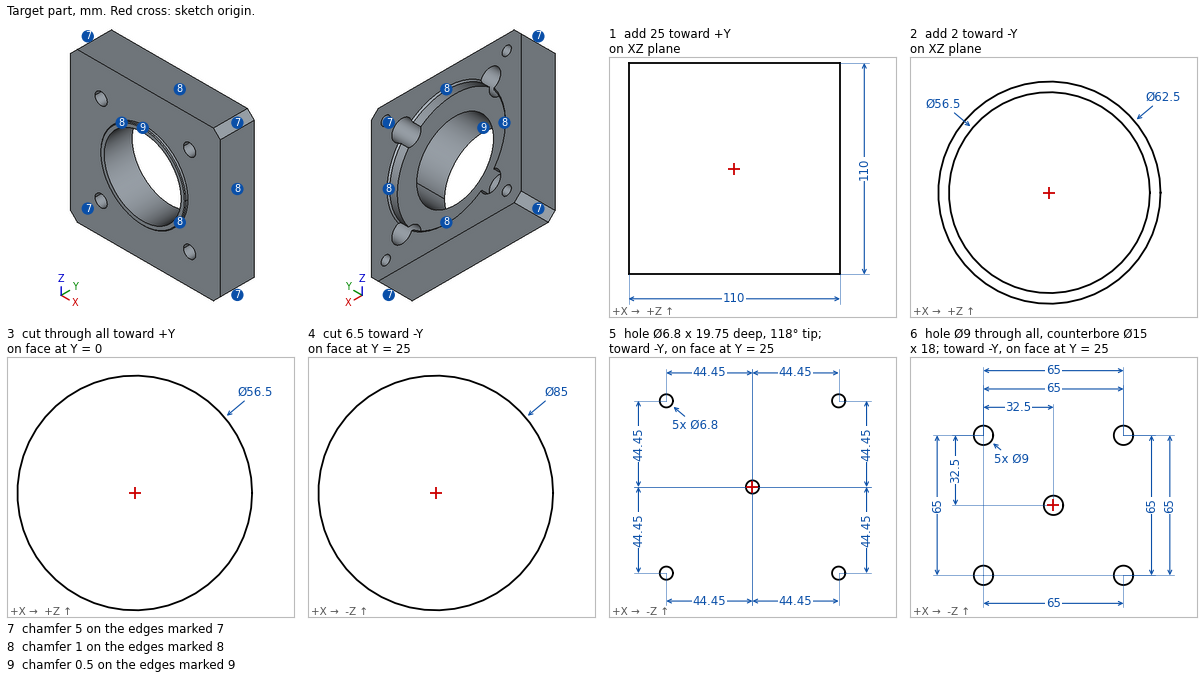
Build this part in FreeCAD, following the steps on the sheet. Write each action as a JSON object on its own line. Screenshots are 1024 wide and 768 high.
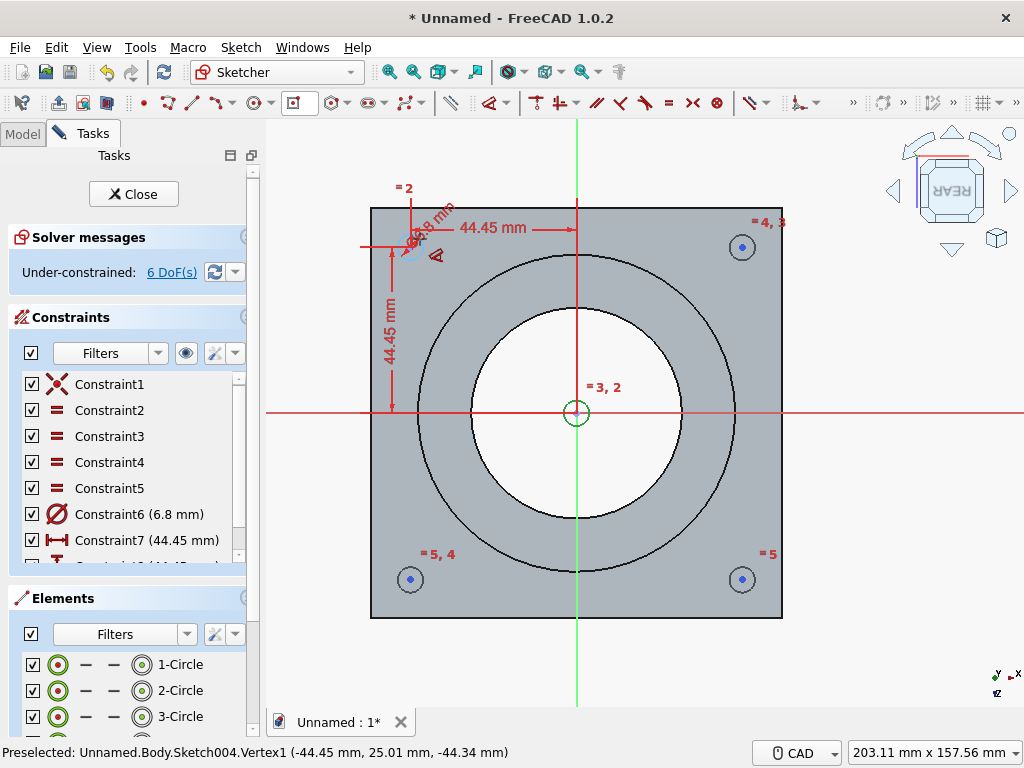
{"action": "left_click", "coordinate": [742, 248]}
{"action": "left_click", "coordinate": [659, 214]}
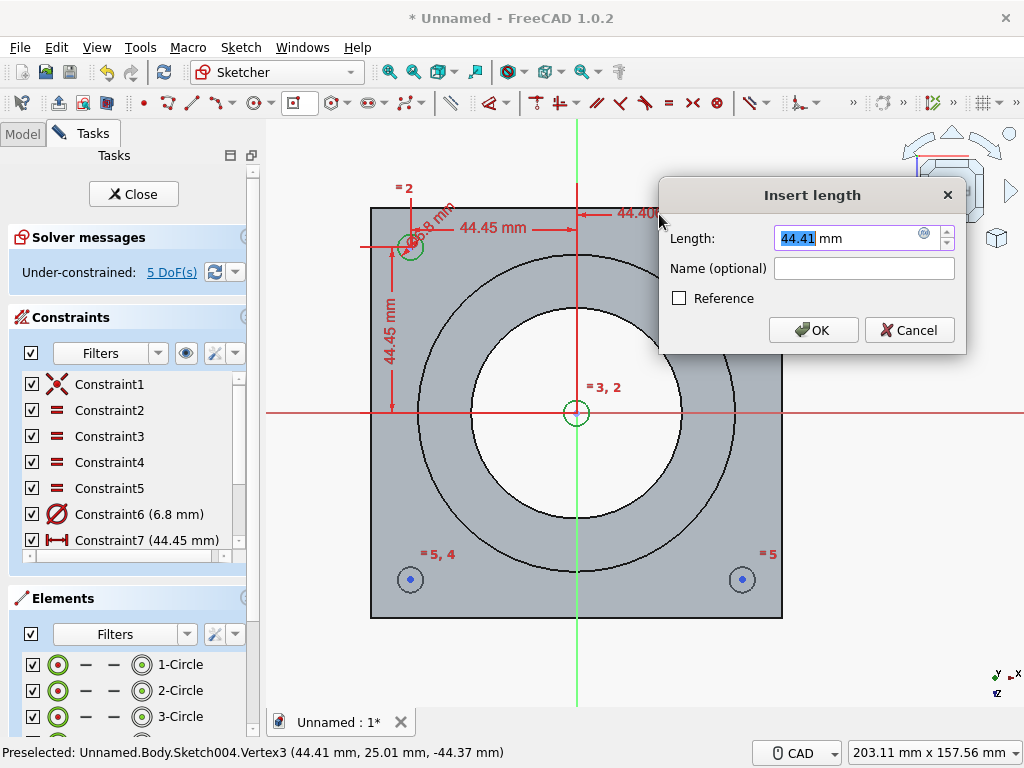
{"action": "type", "text": "44.45"}
{"action": "key", "text": "Return"}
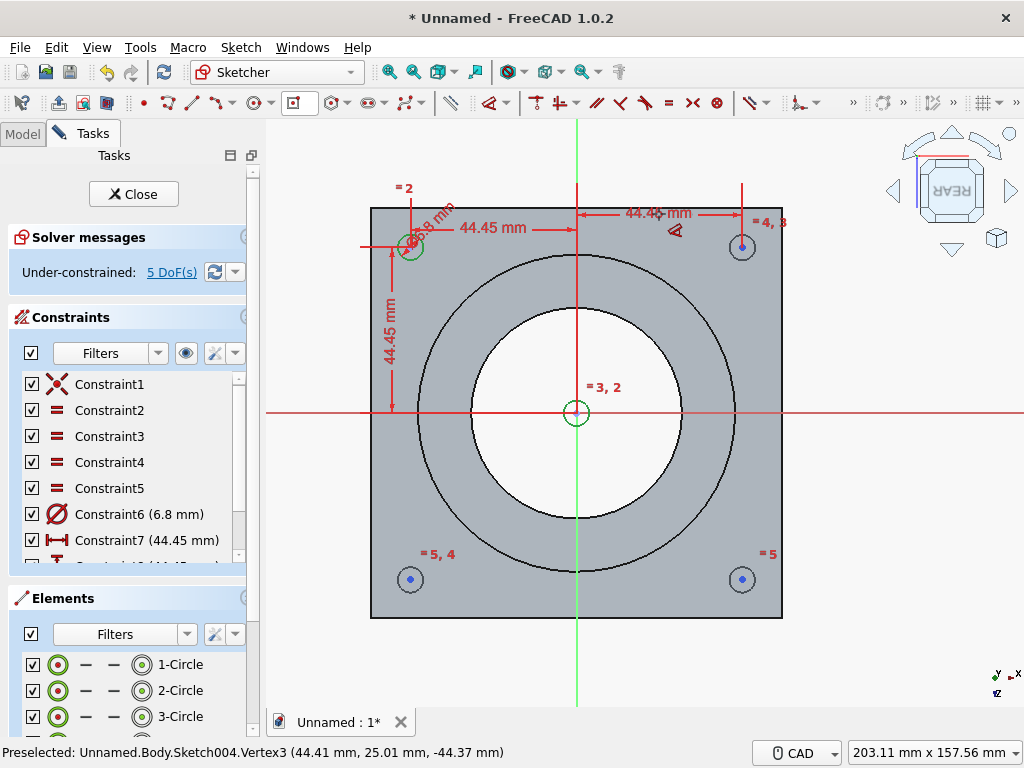
{"action": "left_click", "coordinate": [742, 248]}
{"action": "left_click", "coordinate": [776, 330]}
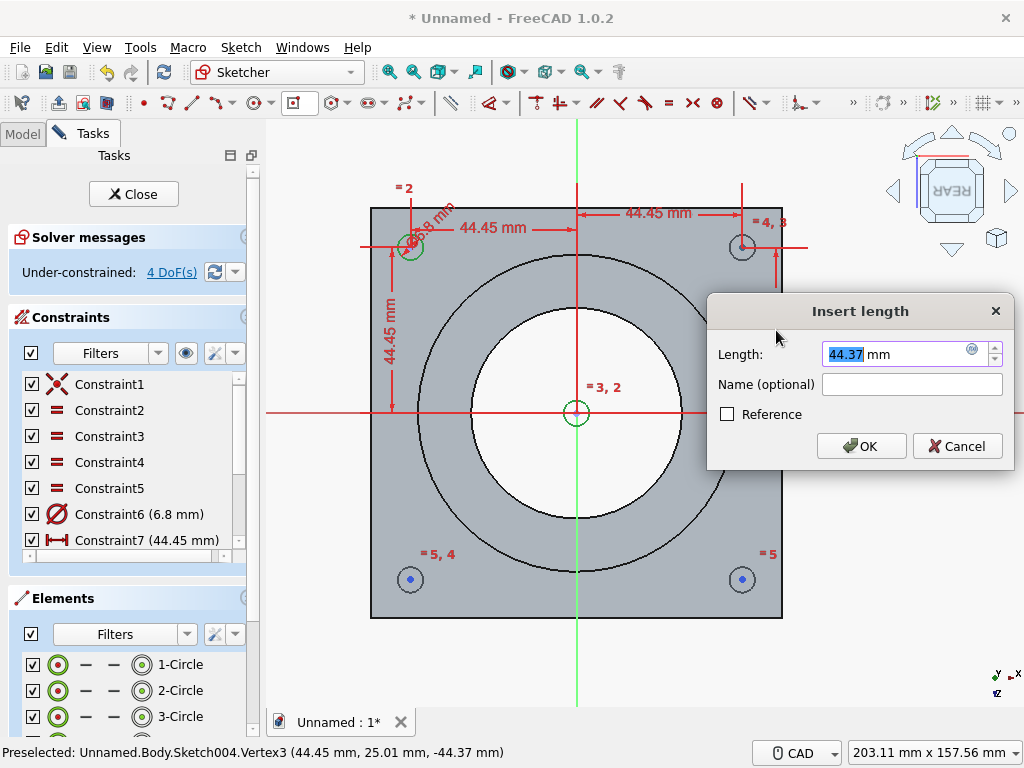
{"action": "type", "text": "44.45"}
{"action": "key", "text": "Return"}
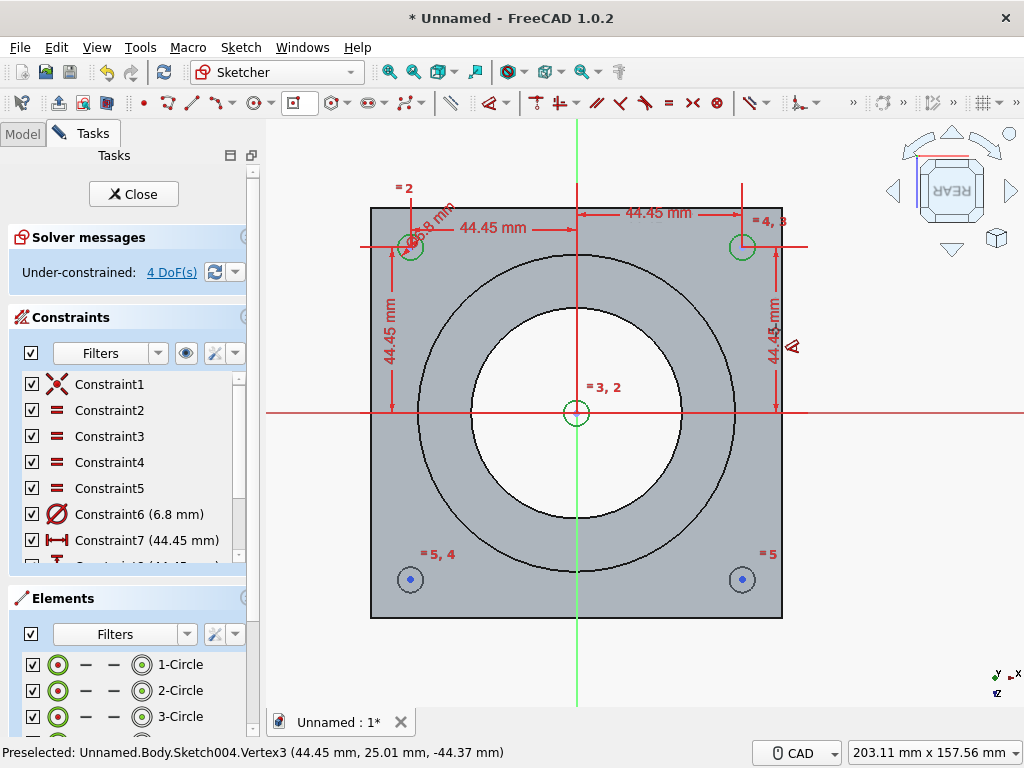
{"action": "left_click", "coordinate": [411, 580]}
{"action": "left_click", "coordinate": [494, 614]}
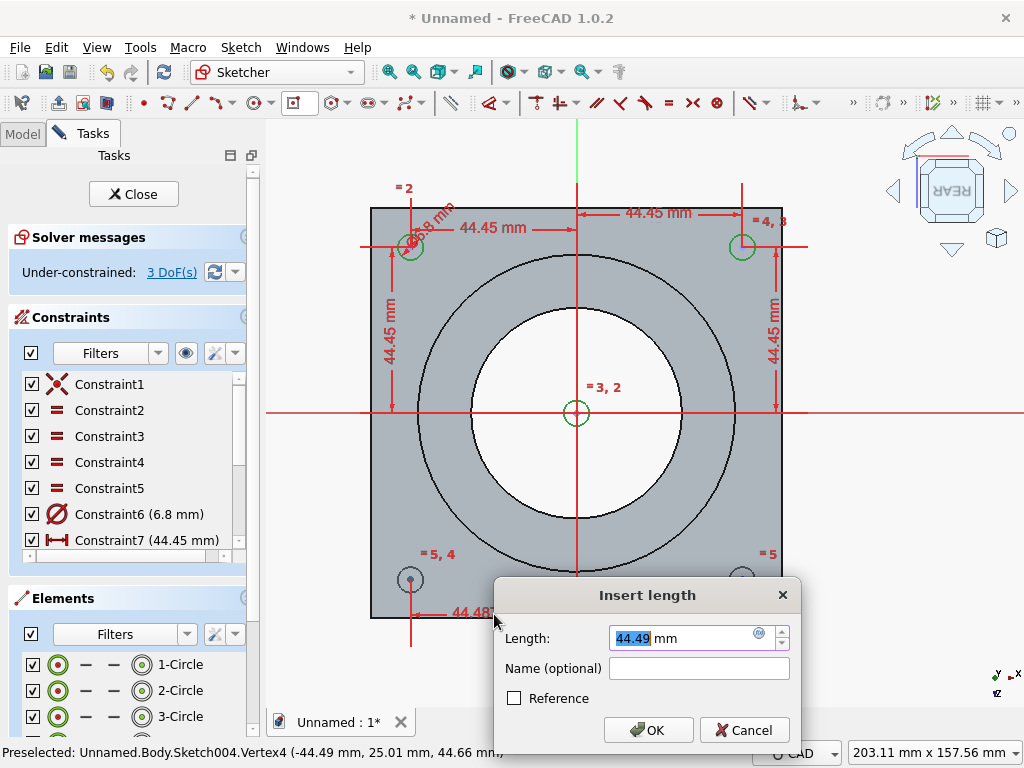
{"action": "type", "text": "44.45"}
{"action": "key", "text": "Return"}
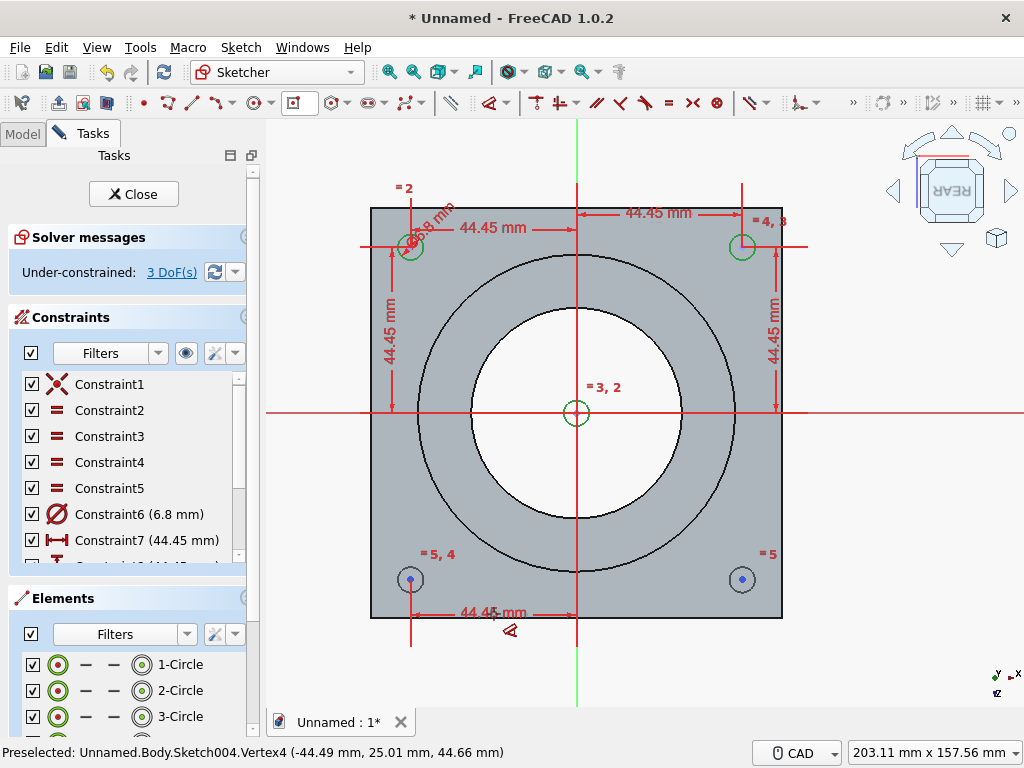
{"action": "left_click", "coordinate": [411, 580]}
{"action": "left_click", "coordinate": [377, 497]}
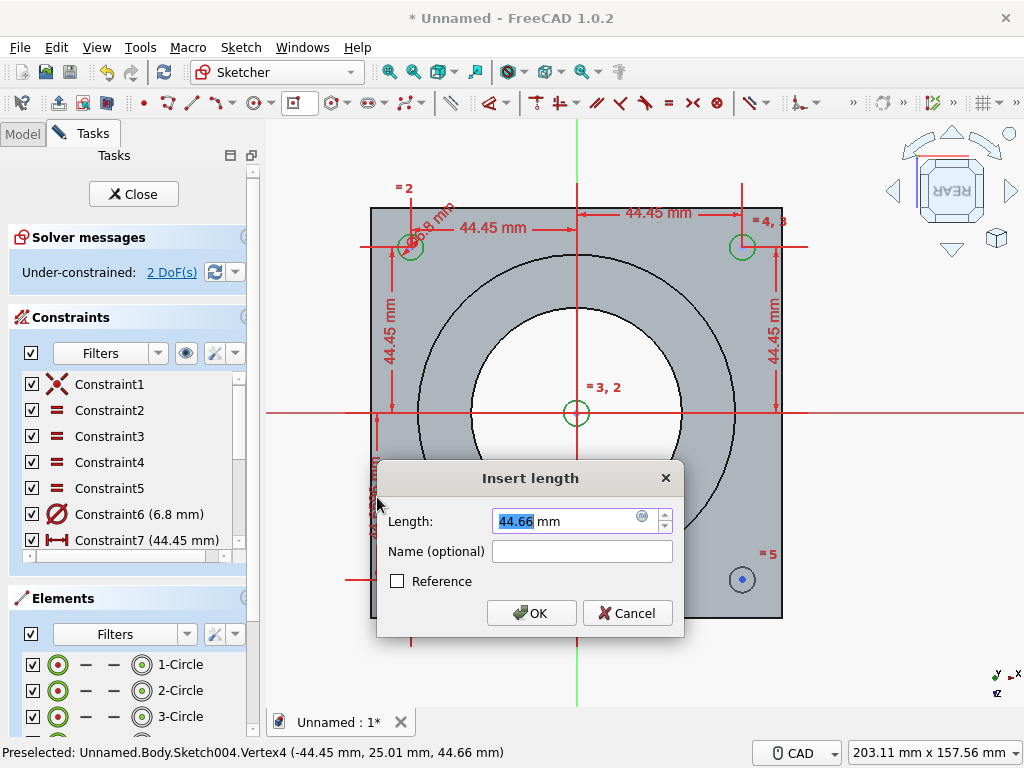
{"action": "type", "text": "44.45"}
{"action": "key", "text": "Return"}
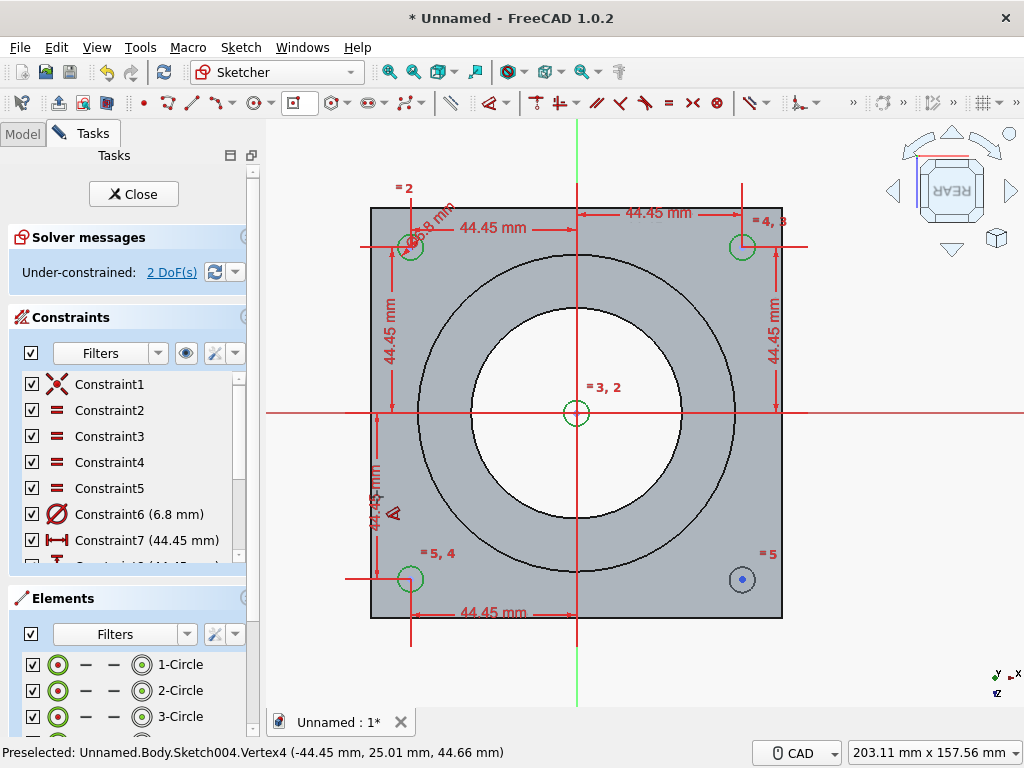
{"action": "left_click", "coordinate": [742, 580]}
{"action": "left_click", "coordinate": [659, 614]}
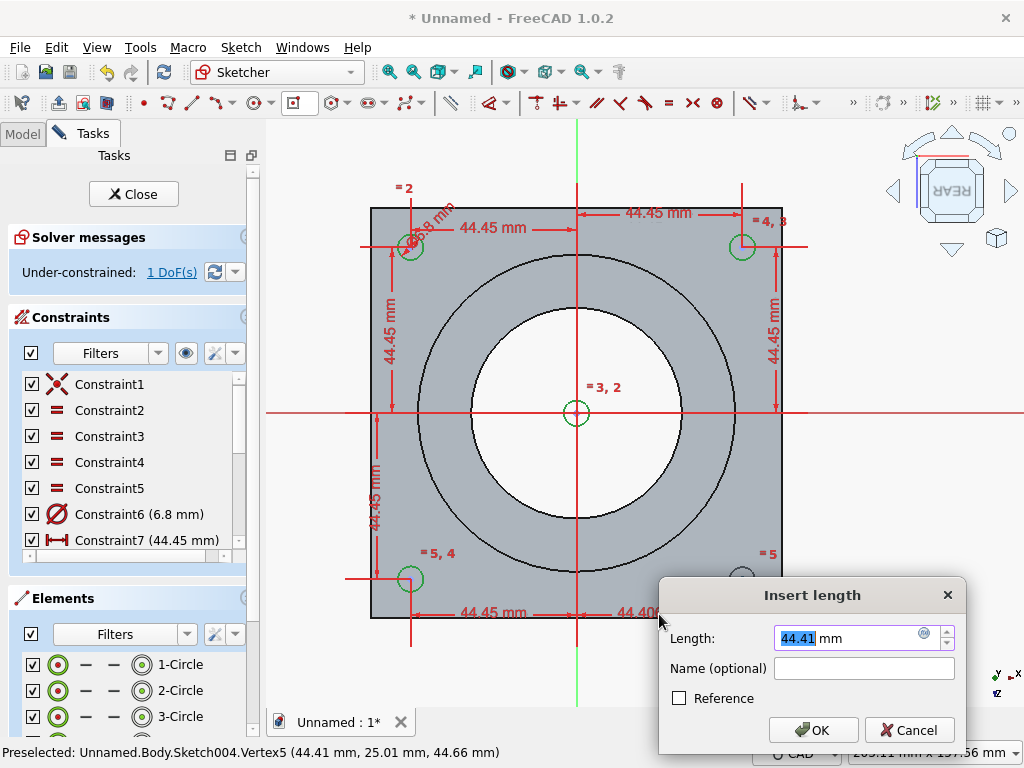
{"action": "type", "text": "44.45"}
{"action": "key", "text": "Return"}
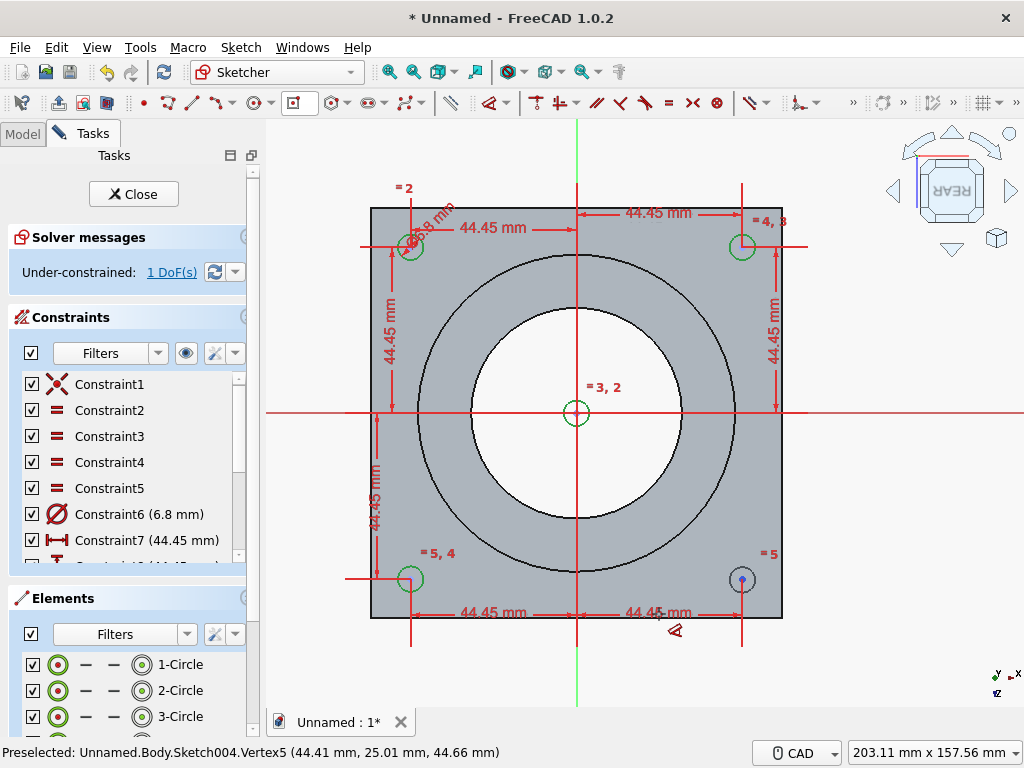
{"action": "left_click", "coordinate": [742, 580]}
{"action": "left_click", "coordinate": [776, 497]}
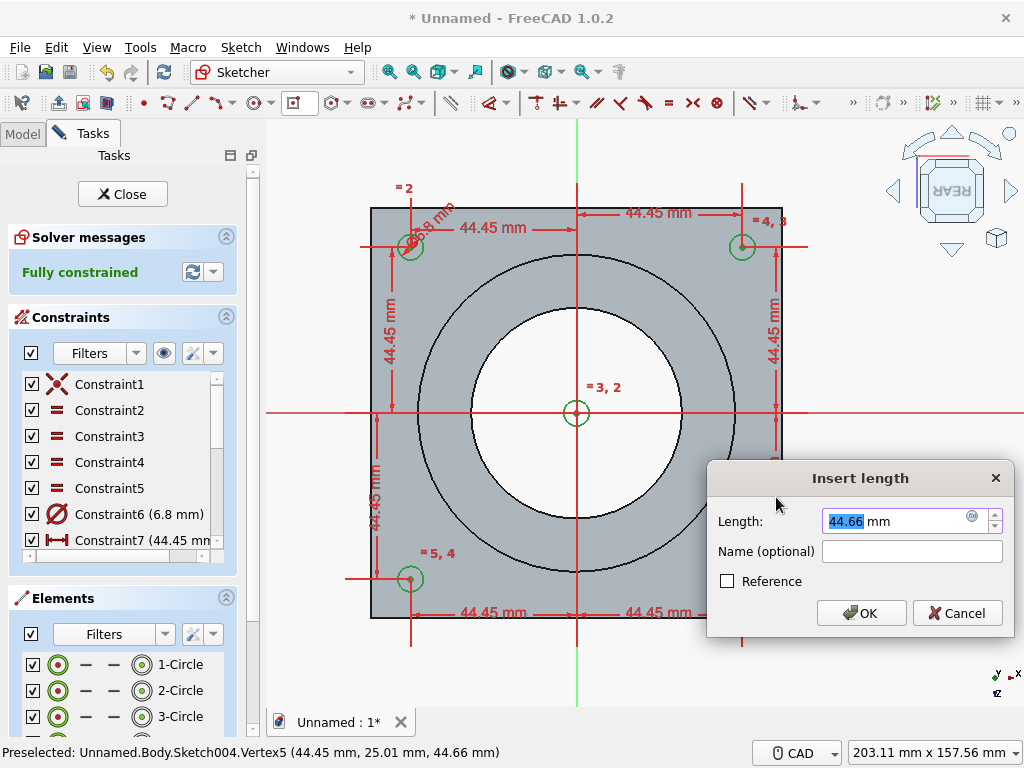
{"action": "type", "text": "44.45"}
{"action": "key", "text": "Return"}
{"action": "key", "text": "Escape"}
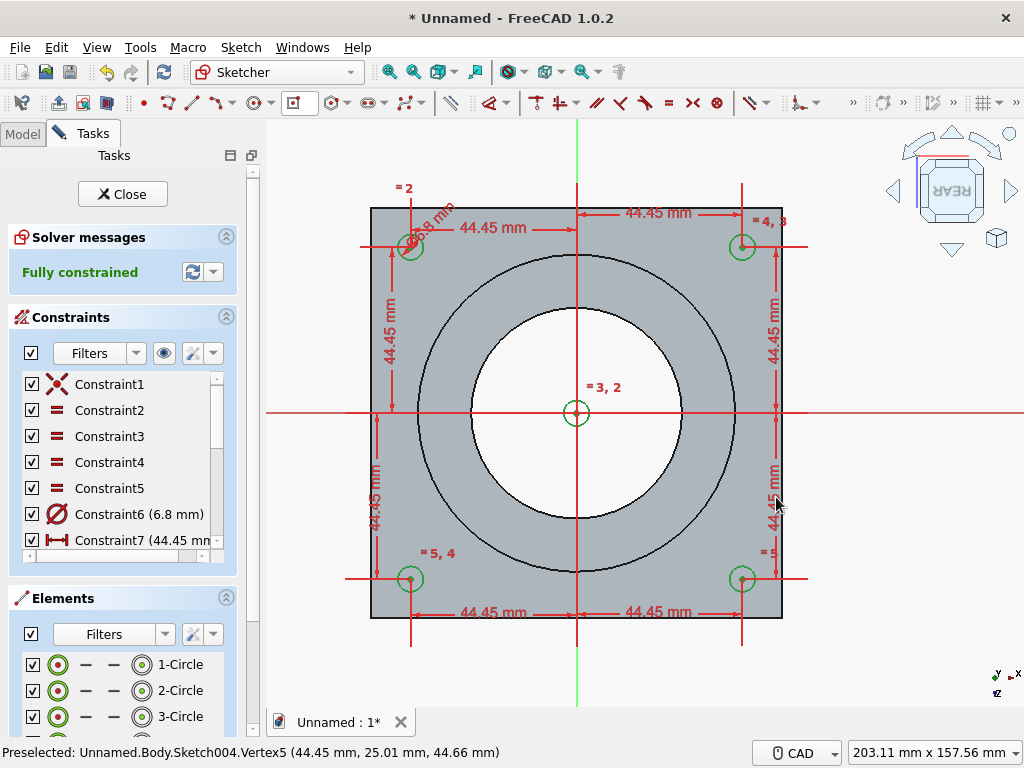
{"action": "left_click", "coordinate": [123, 194]}